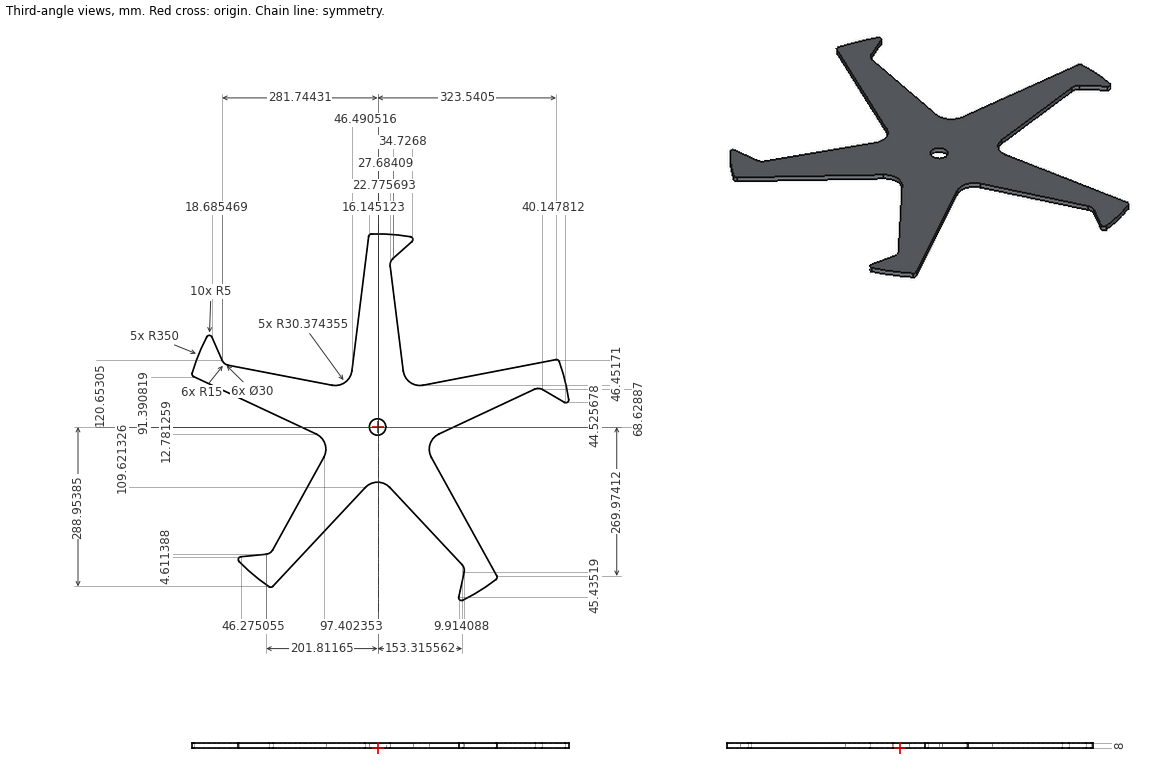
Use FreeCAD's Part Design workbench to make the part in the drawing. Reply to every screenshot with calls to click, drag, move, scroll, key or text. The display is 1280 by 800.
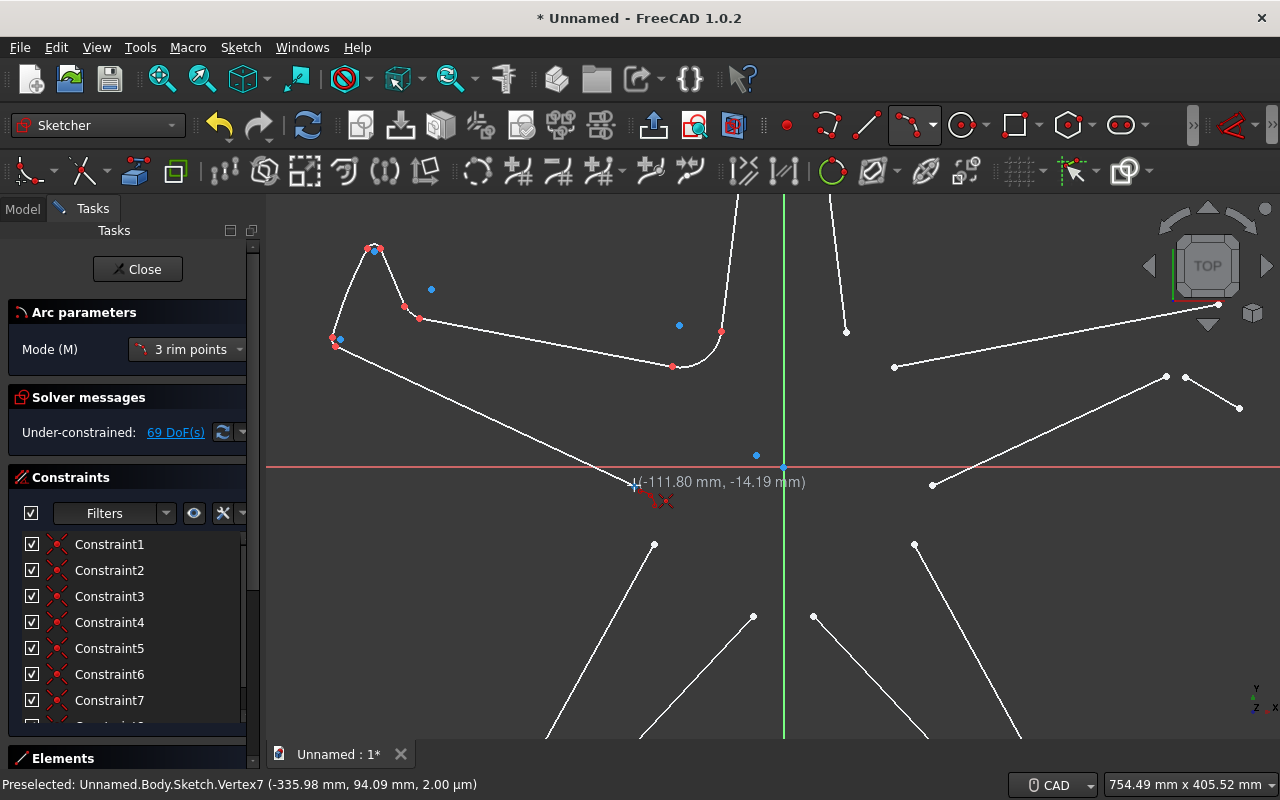
click(635, 486)
click(654, 544)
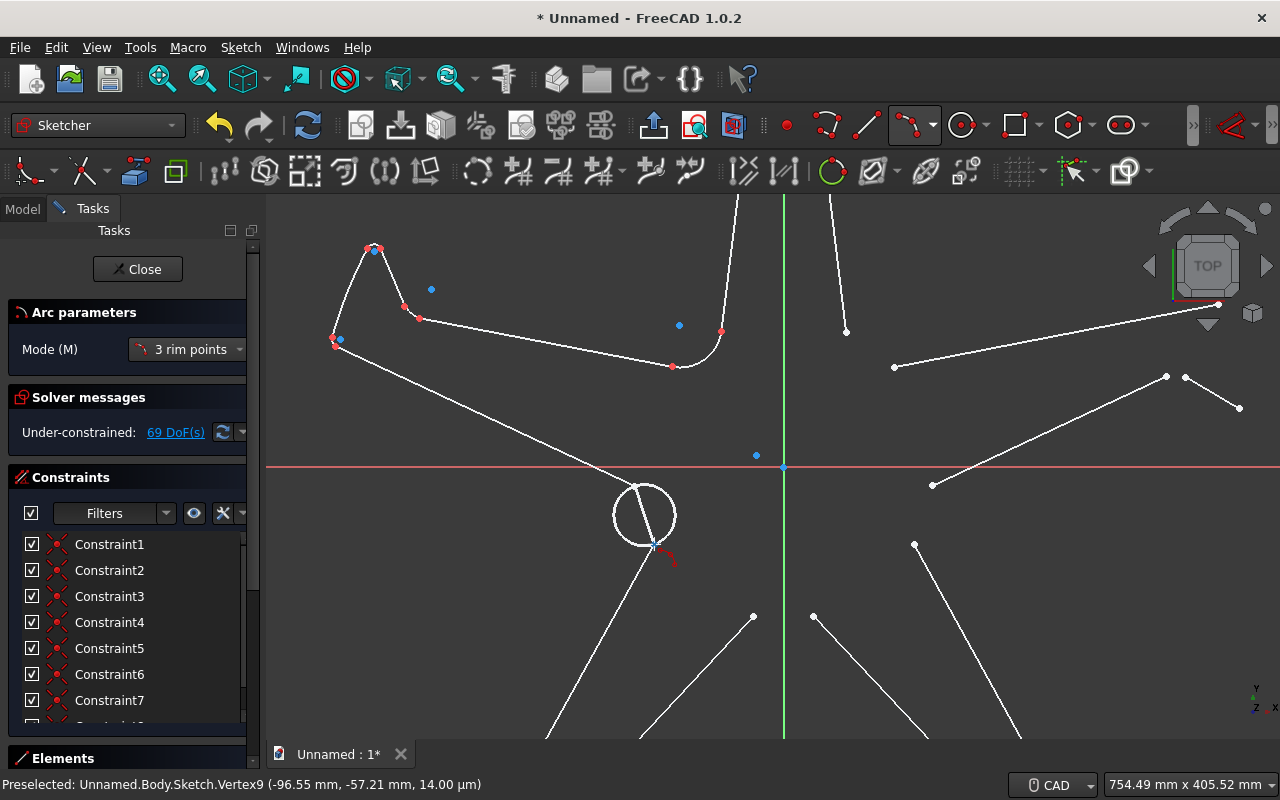
scroll(656, 509, up, 2)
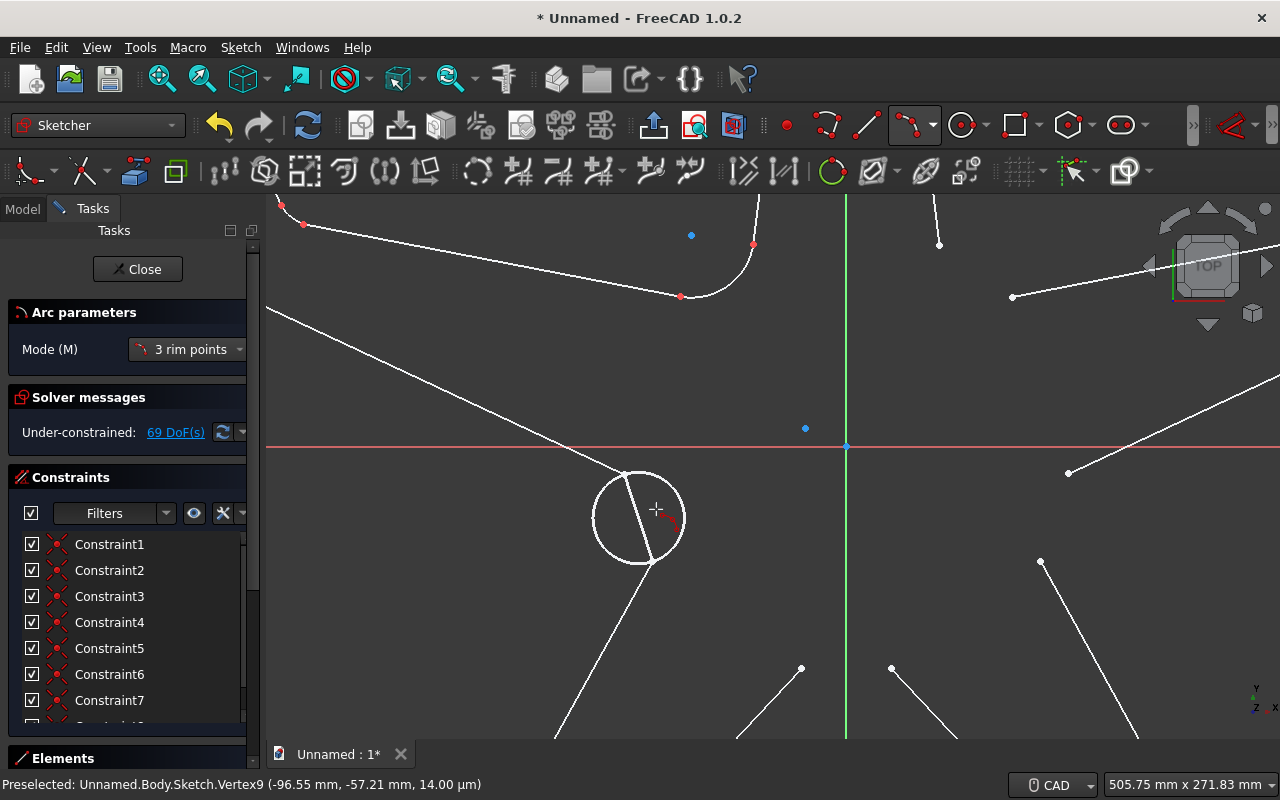
click(656, 509)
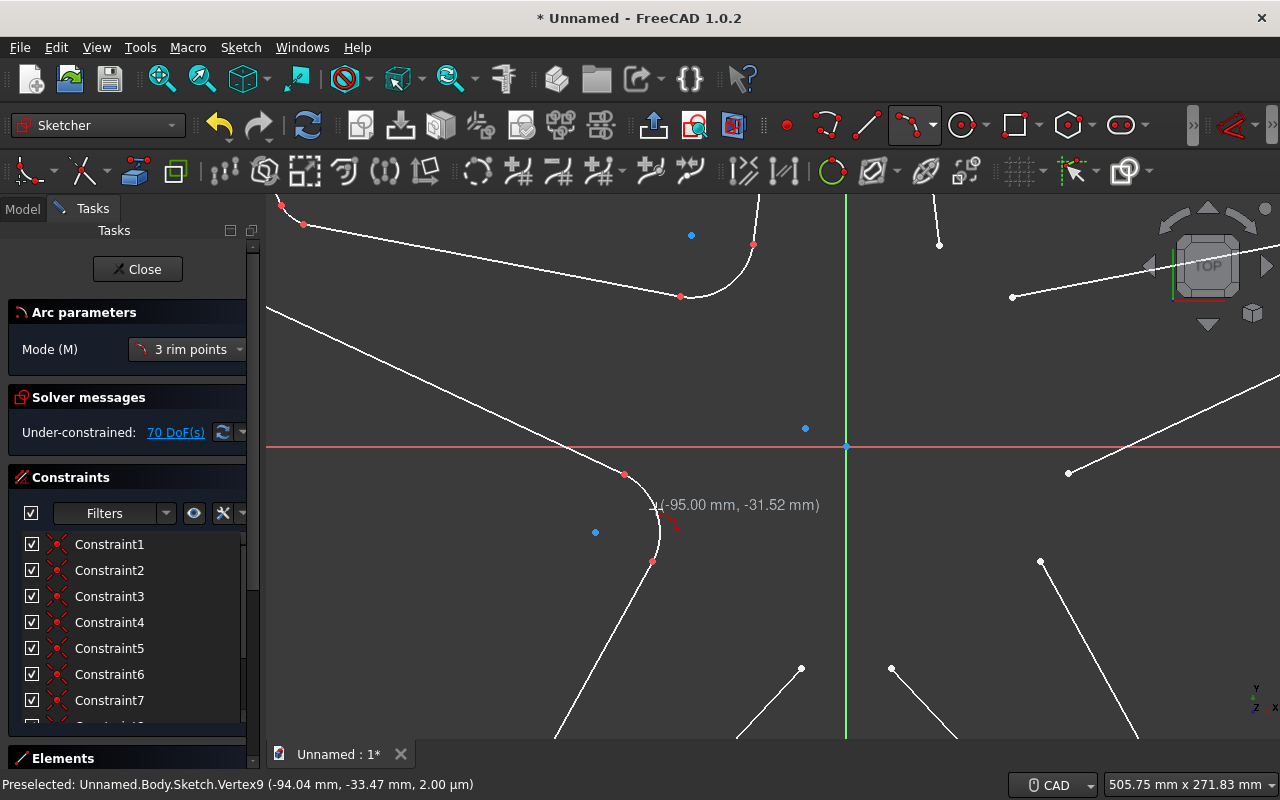
scroll(655, 485, down, 7)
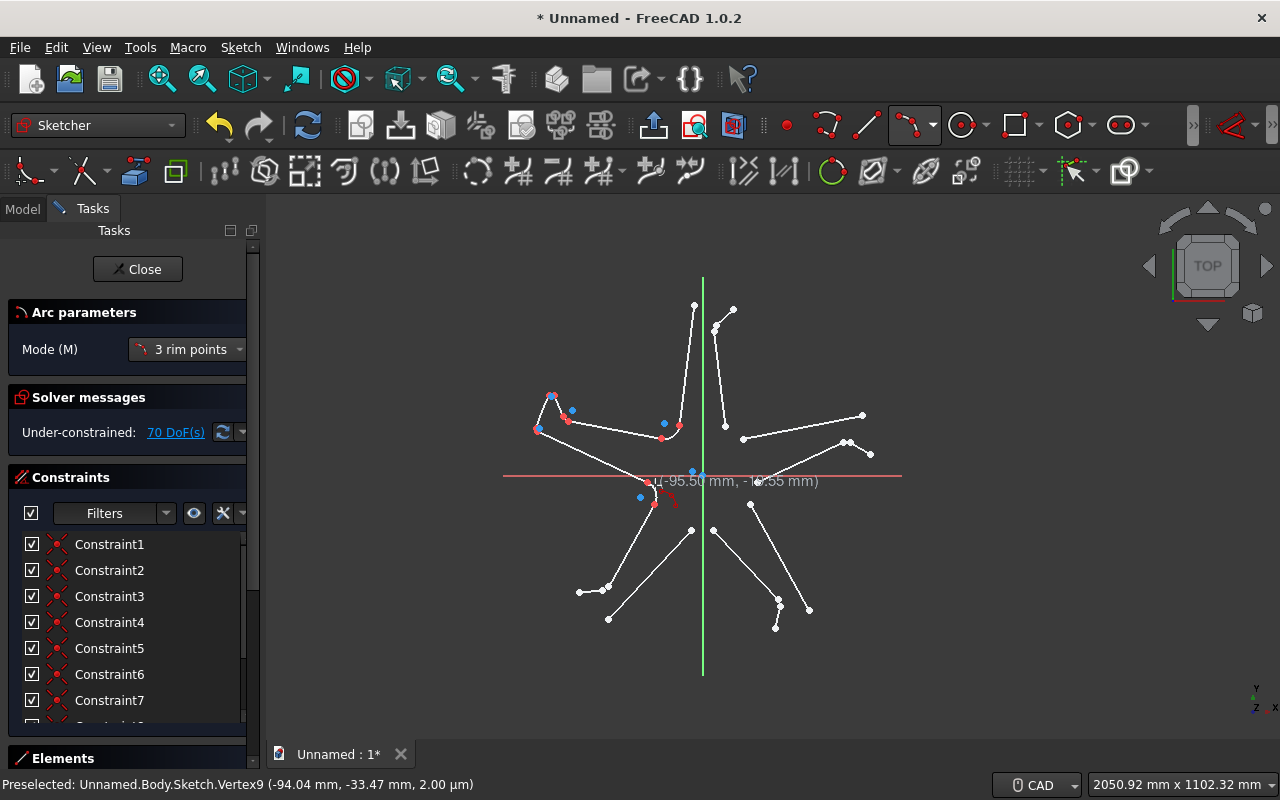
scroll(608, 586, up, 5)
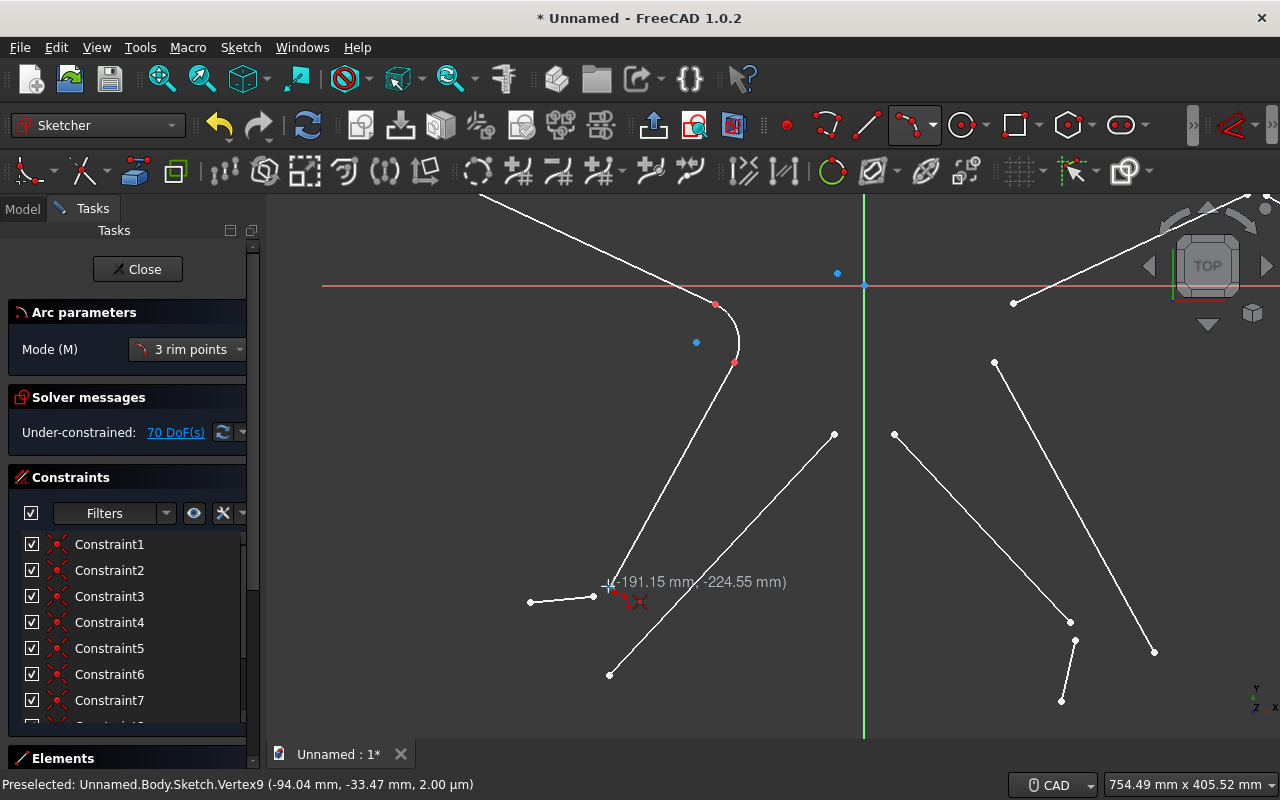
click(610, 587)
click(593, 597)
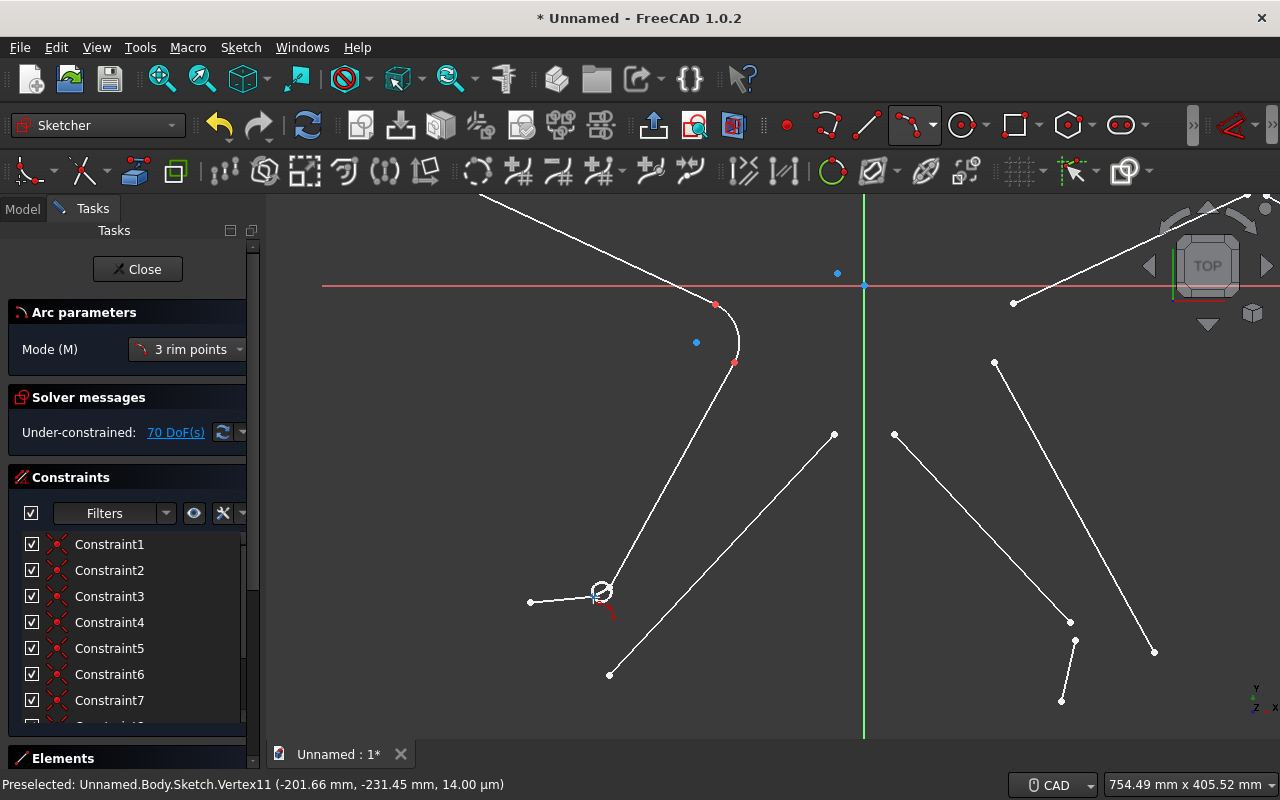
scroll(602, 592, up, 10)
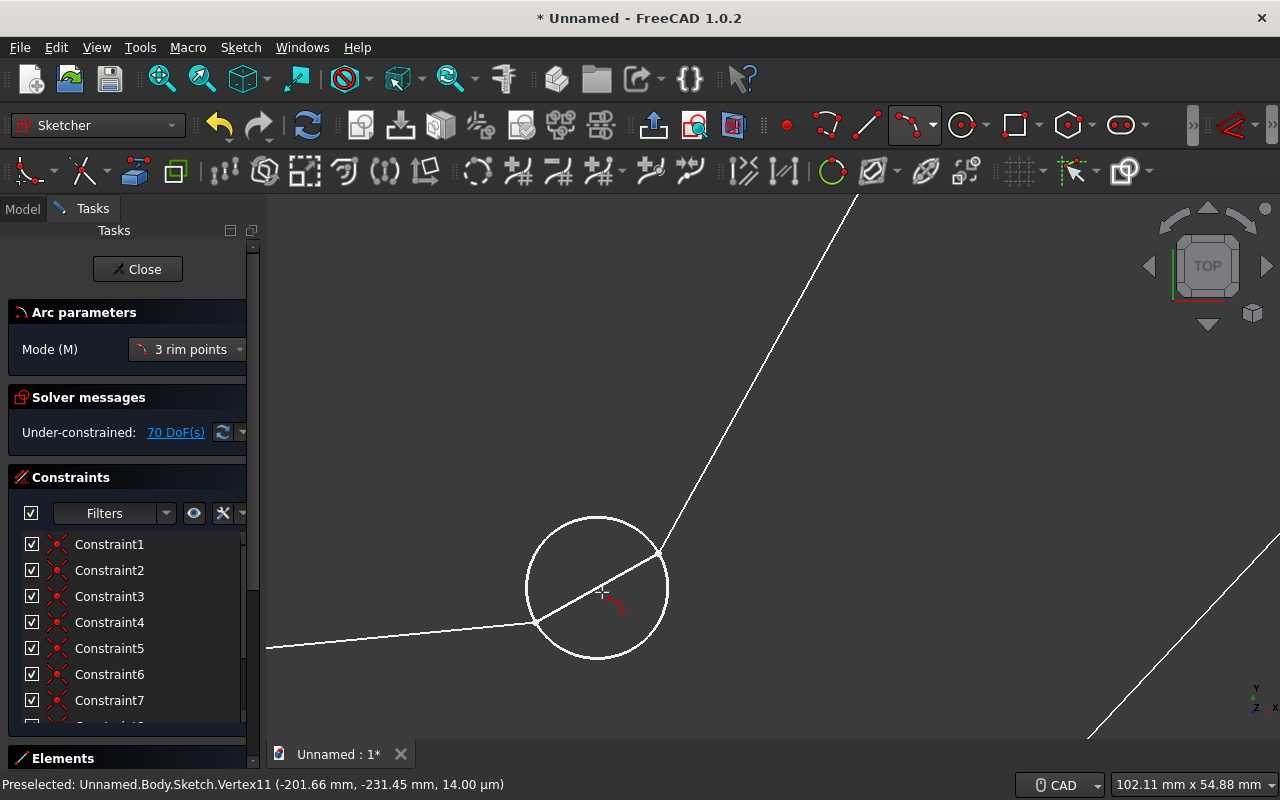
click(601, 591)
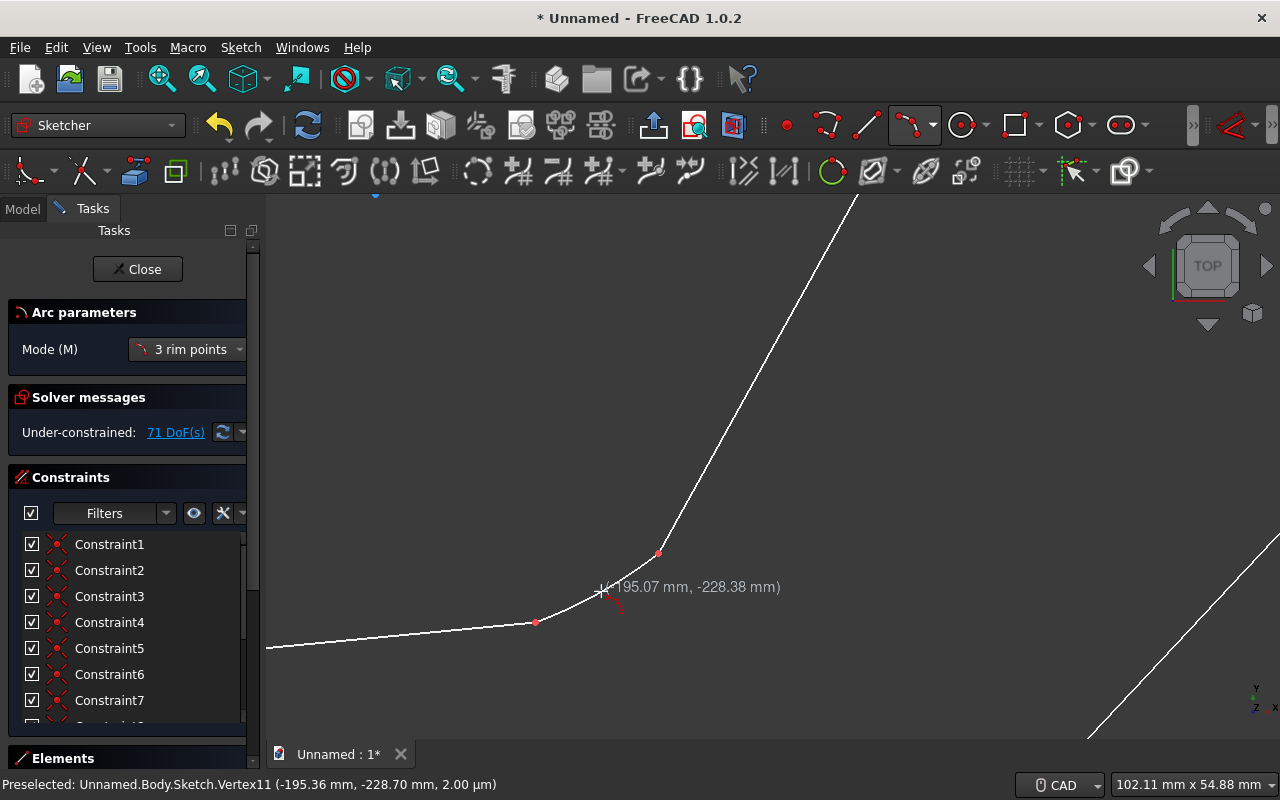
scroll(606, 588, down, 15)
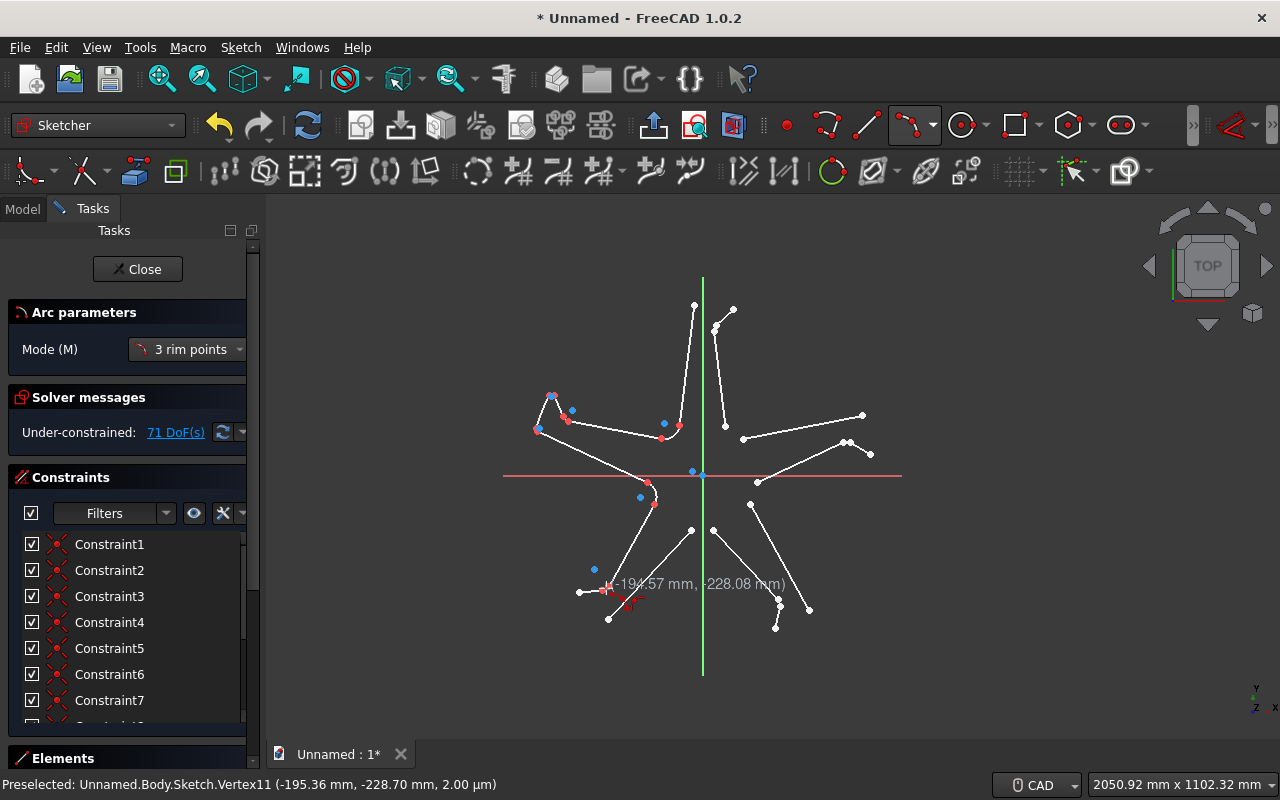
scroll(580, 592, up, 2)